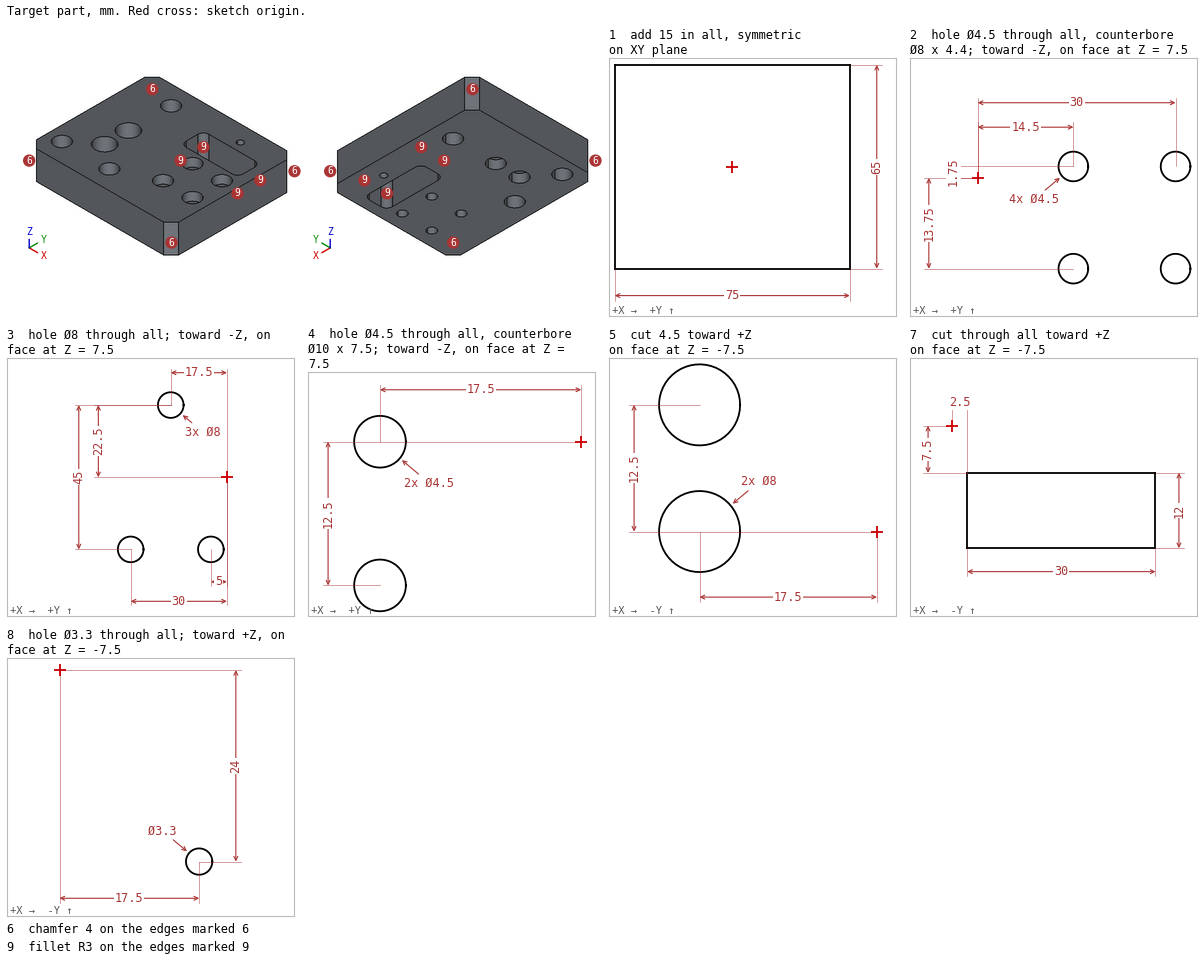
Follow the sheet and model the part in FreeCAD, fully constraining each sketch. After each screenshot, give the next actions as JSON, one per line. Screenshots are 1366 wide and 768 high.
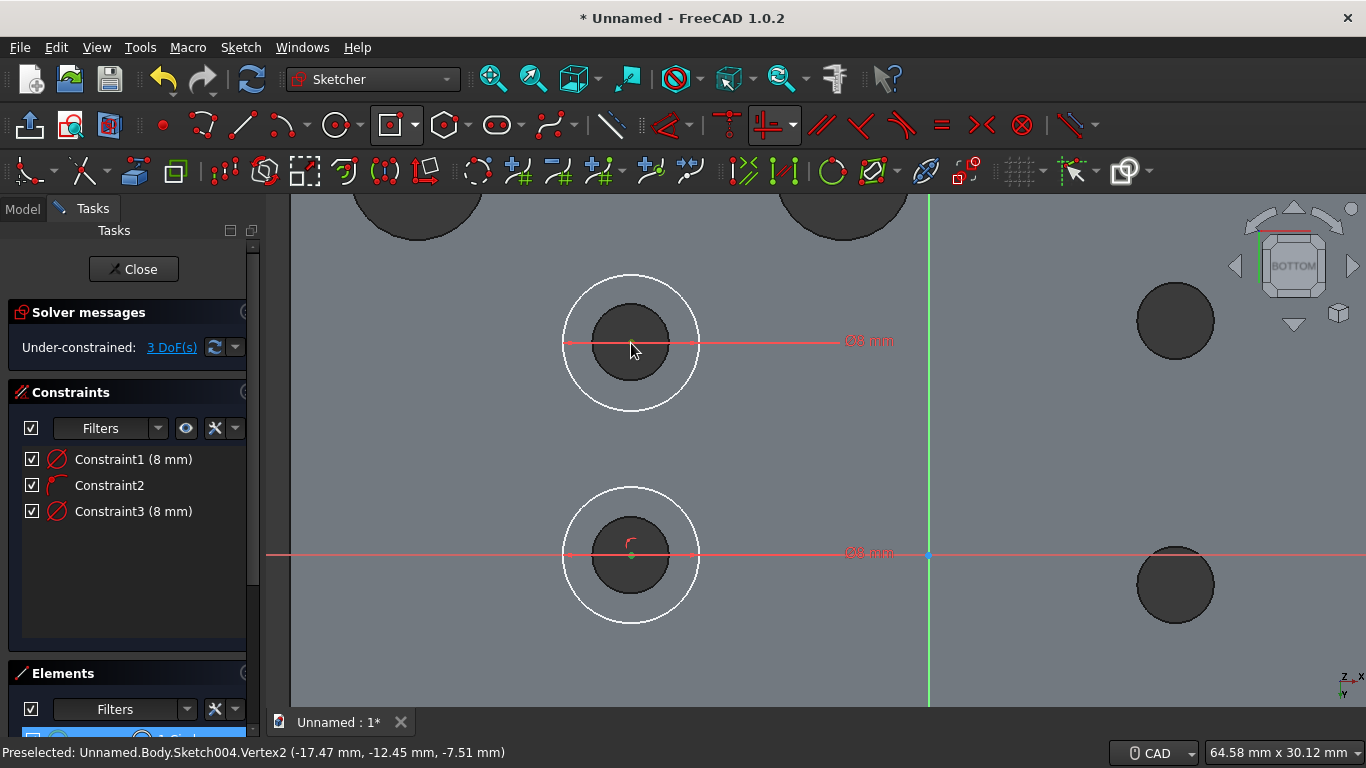
{"action": "key", "text": "v"}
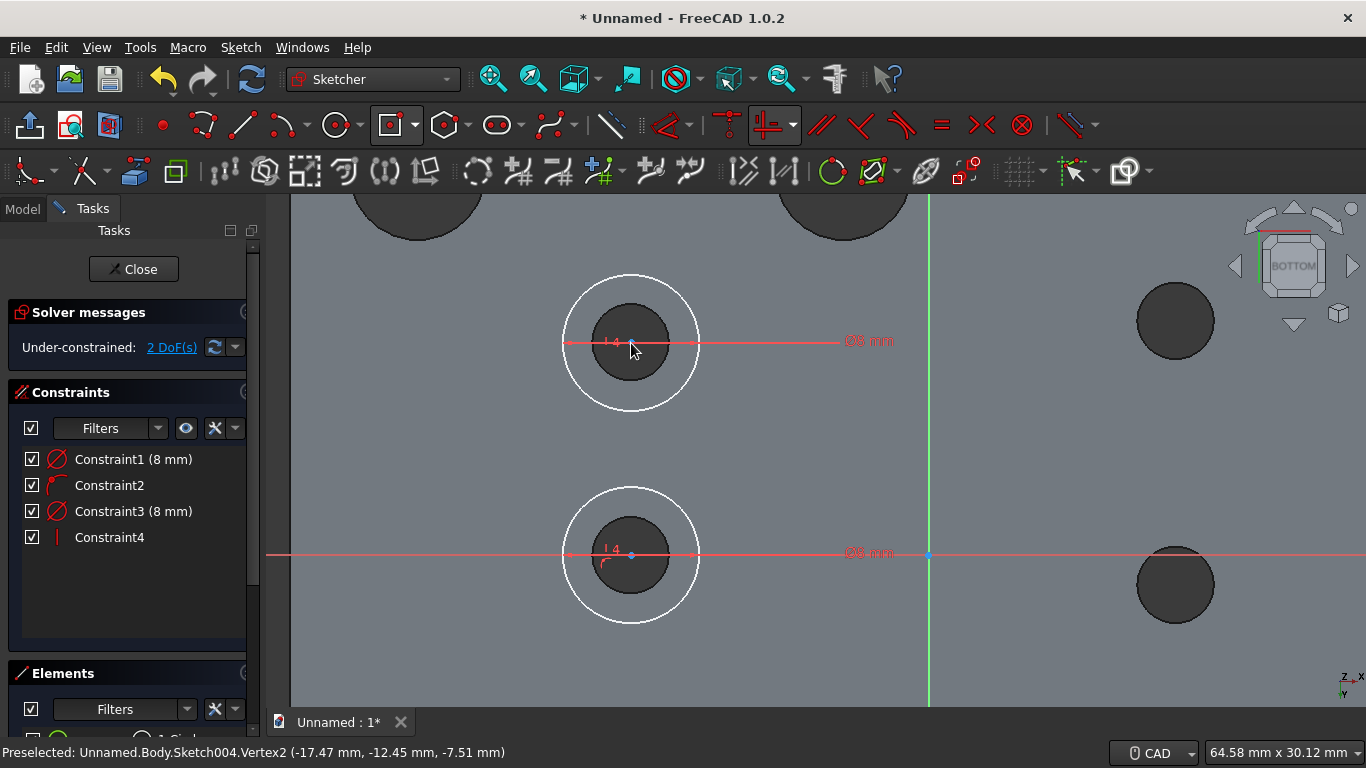
{"action": "left_click", "coordinate": [631, 555]}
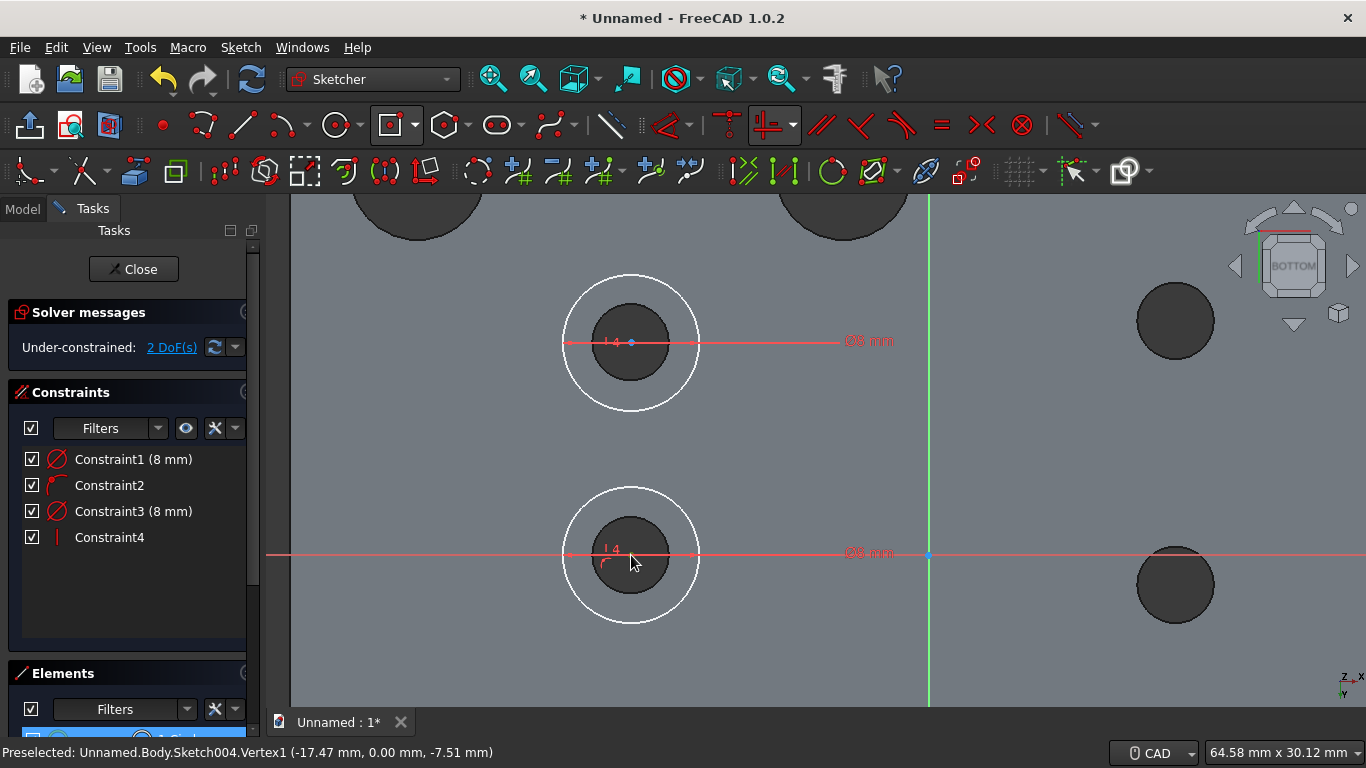
{"action": "key", "text": "l"}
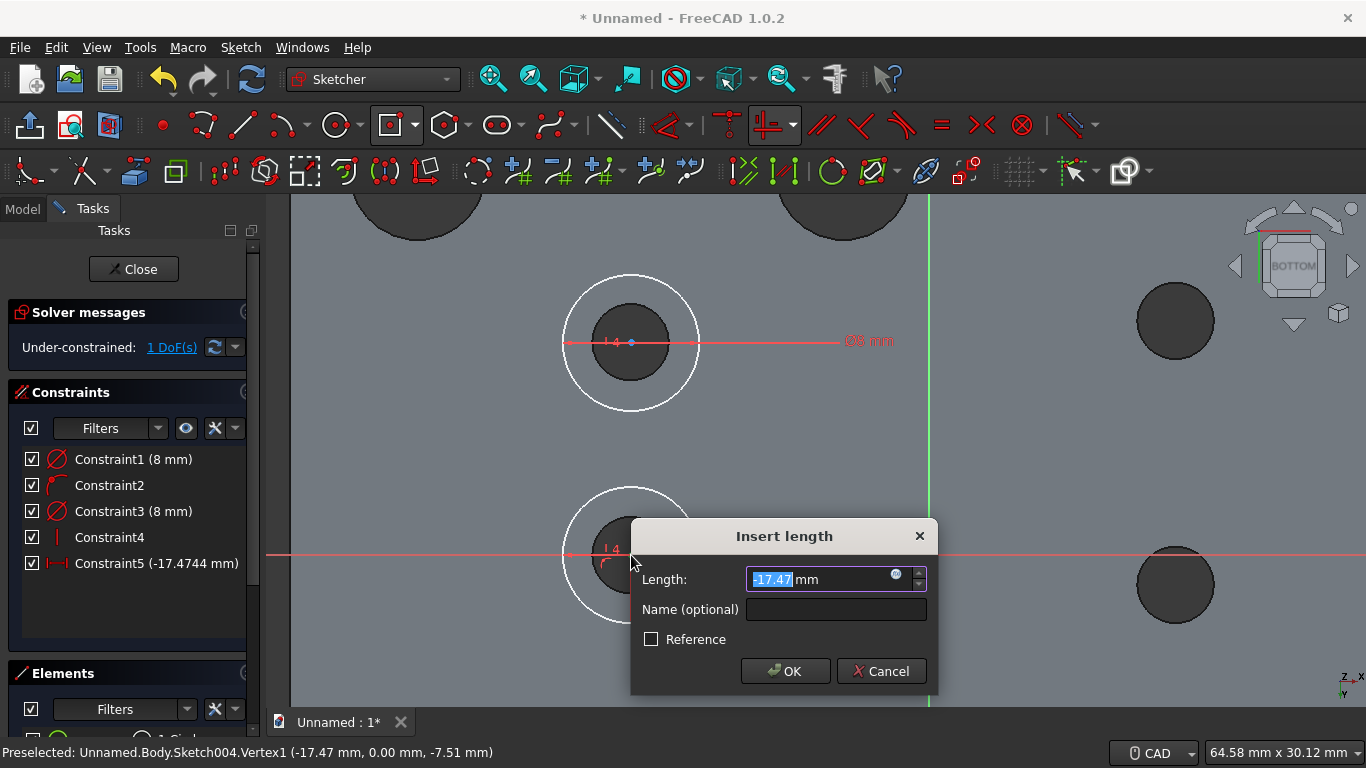
{"action": "type", "text": "-17.5"}
{"action": "key", "text": "Return"}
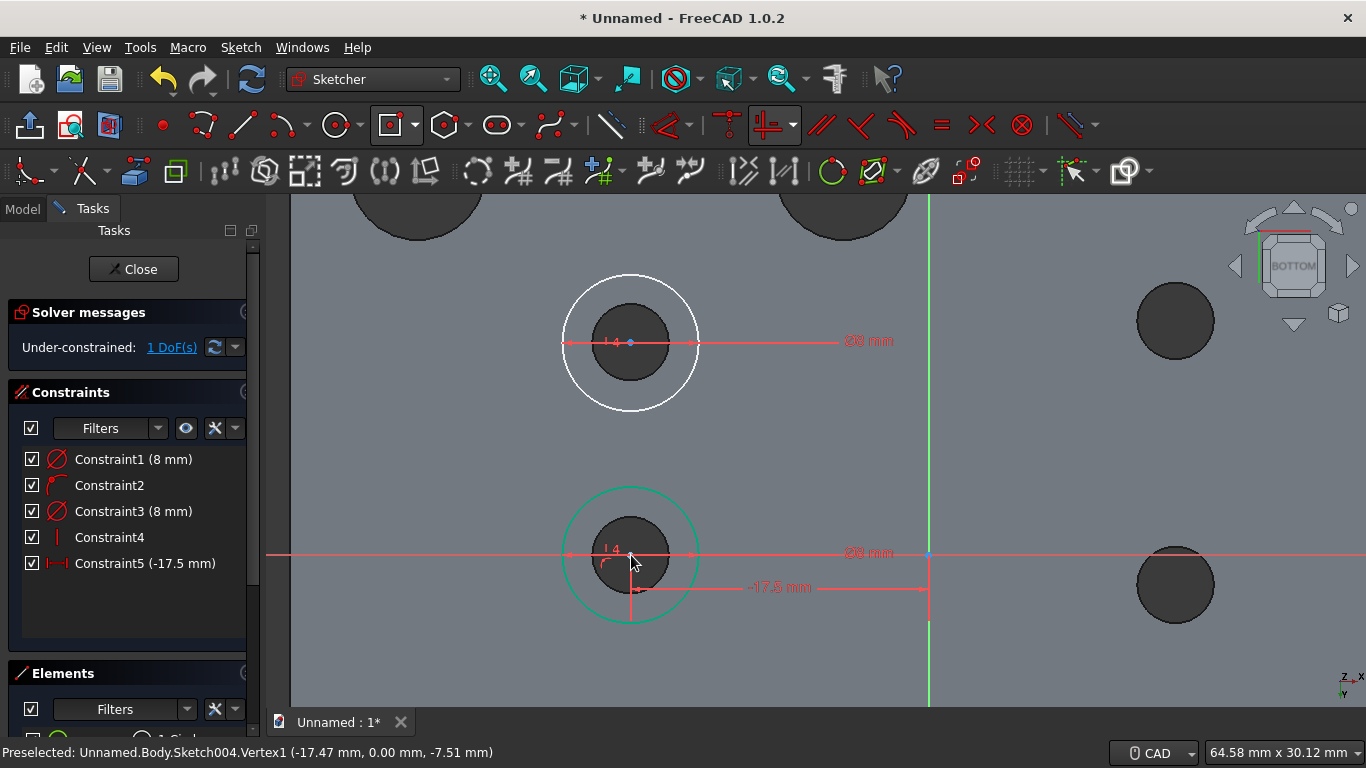
{"action": "left_click", "coordinate": [631, 343]}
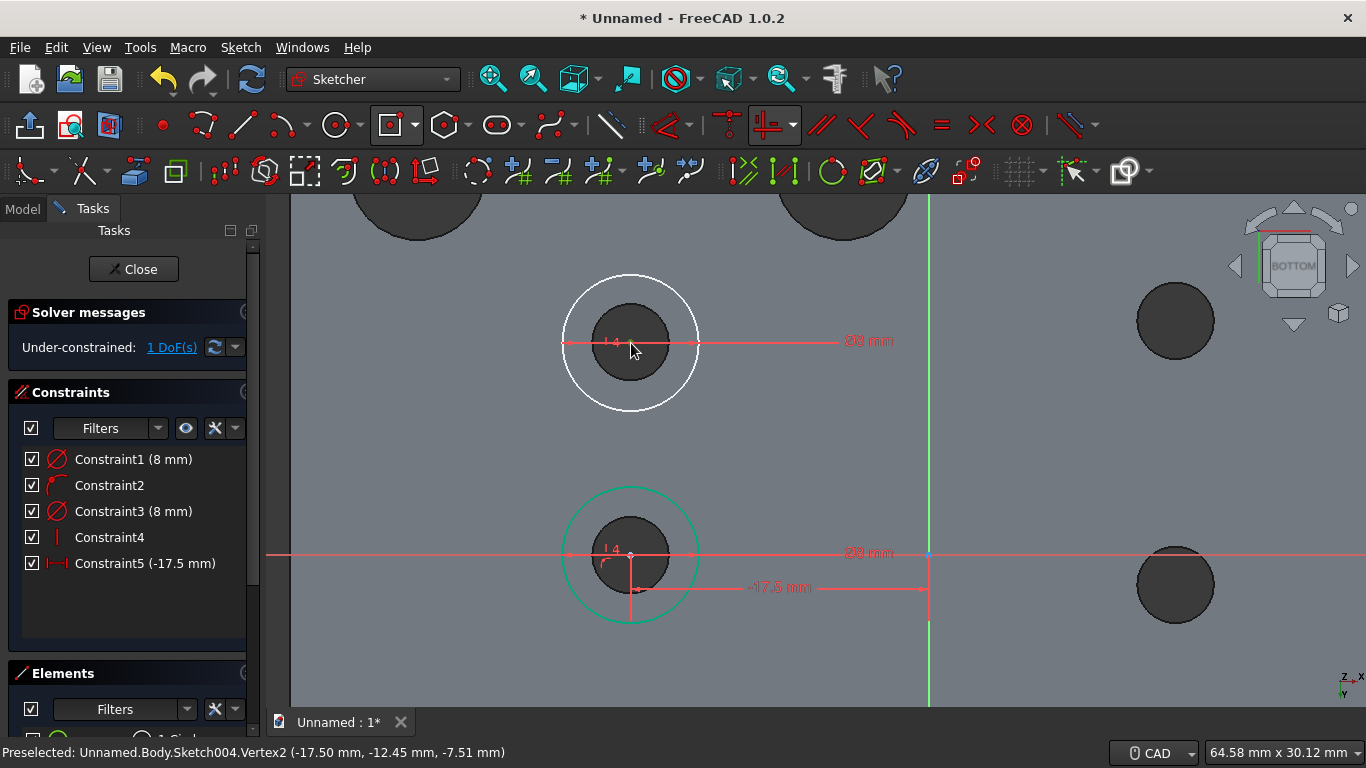
{"action": "key", "text": "i"}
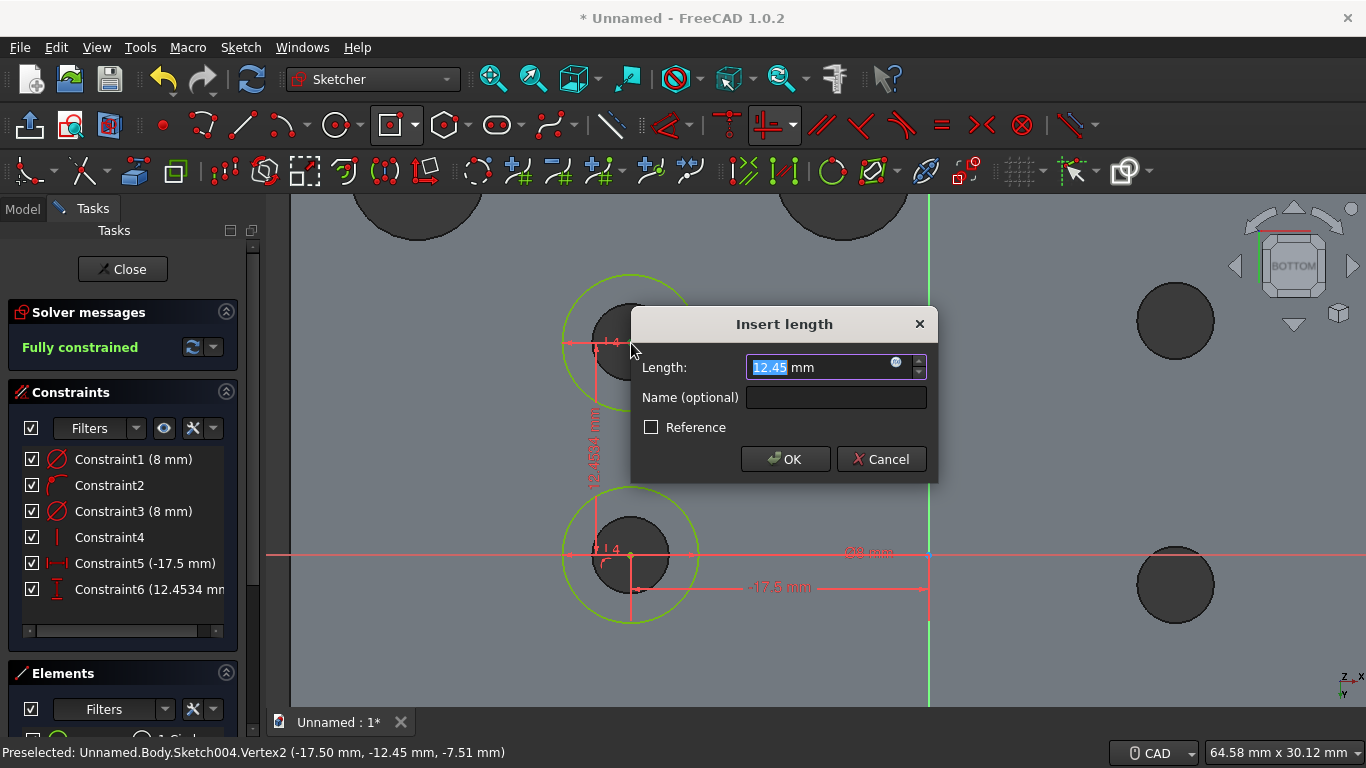
{"action": "type", "text": "12.5"}
{"action": "key", "text": "Return"}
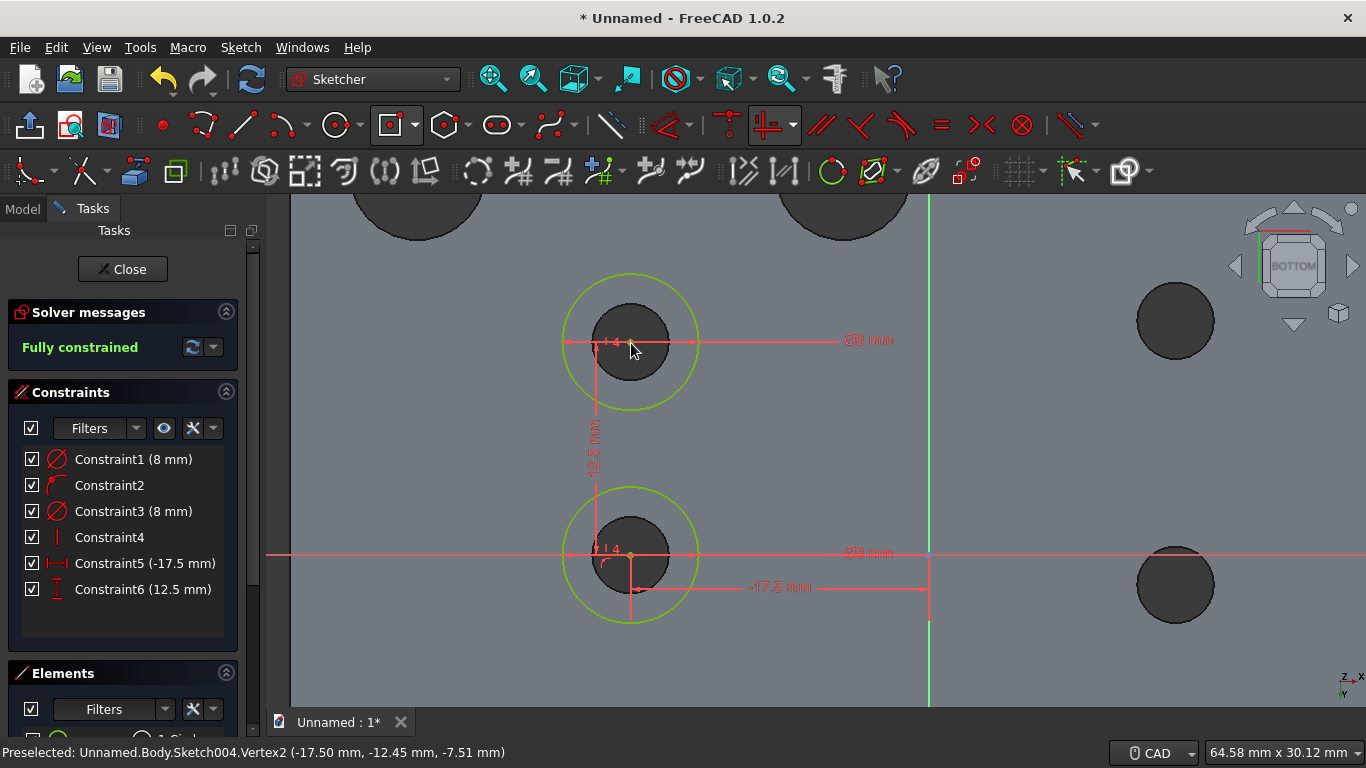
{"action": "left_click", "coordinate": [123, 269]}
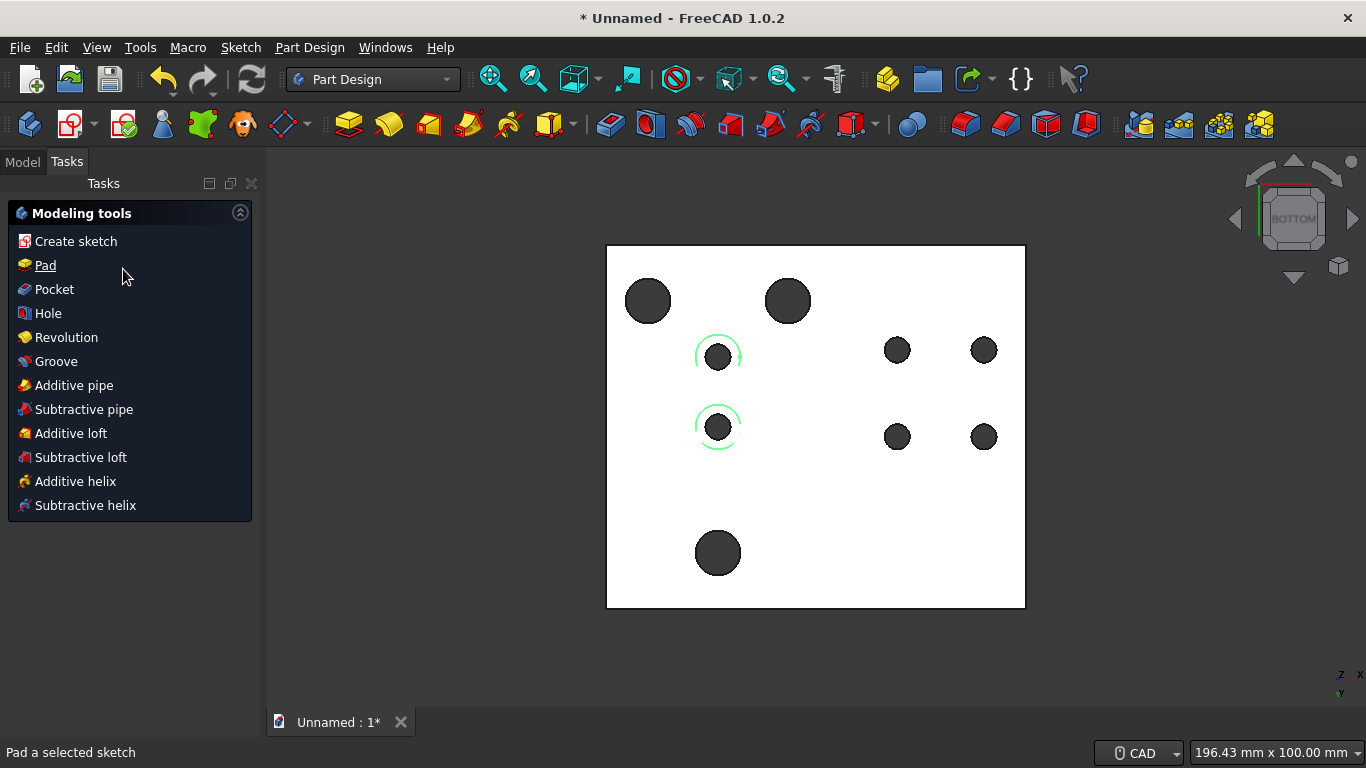
{"action": "left_click", "coordinate": [612, 124]}